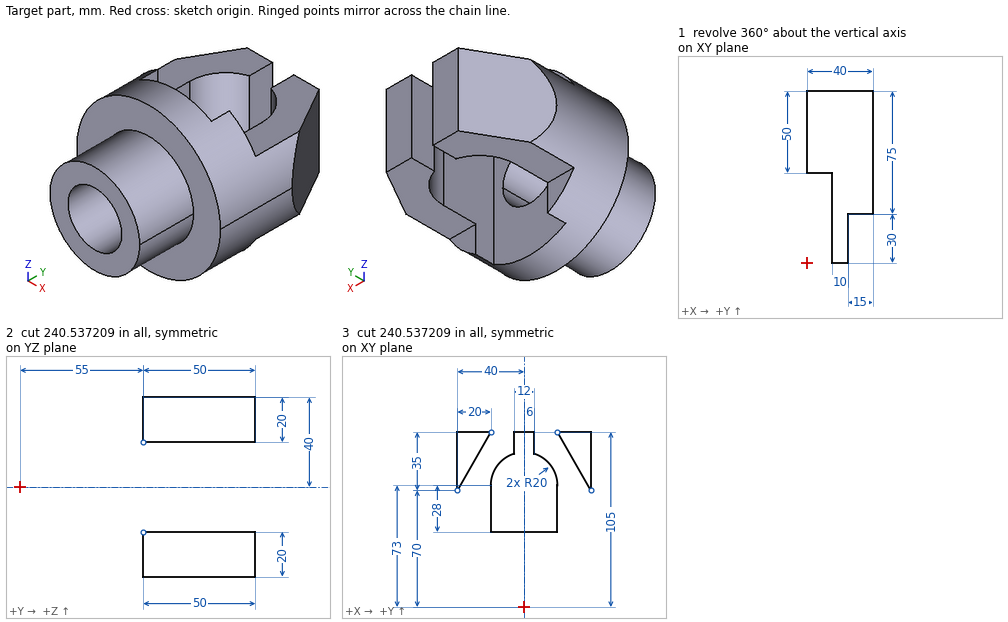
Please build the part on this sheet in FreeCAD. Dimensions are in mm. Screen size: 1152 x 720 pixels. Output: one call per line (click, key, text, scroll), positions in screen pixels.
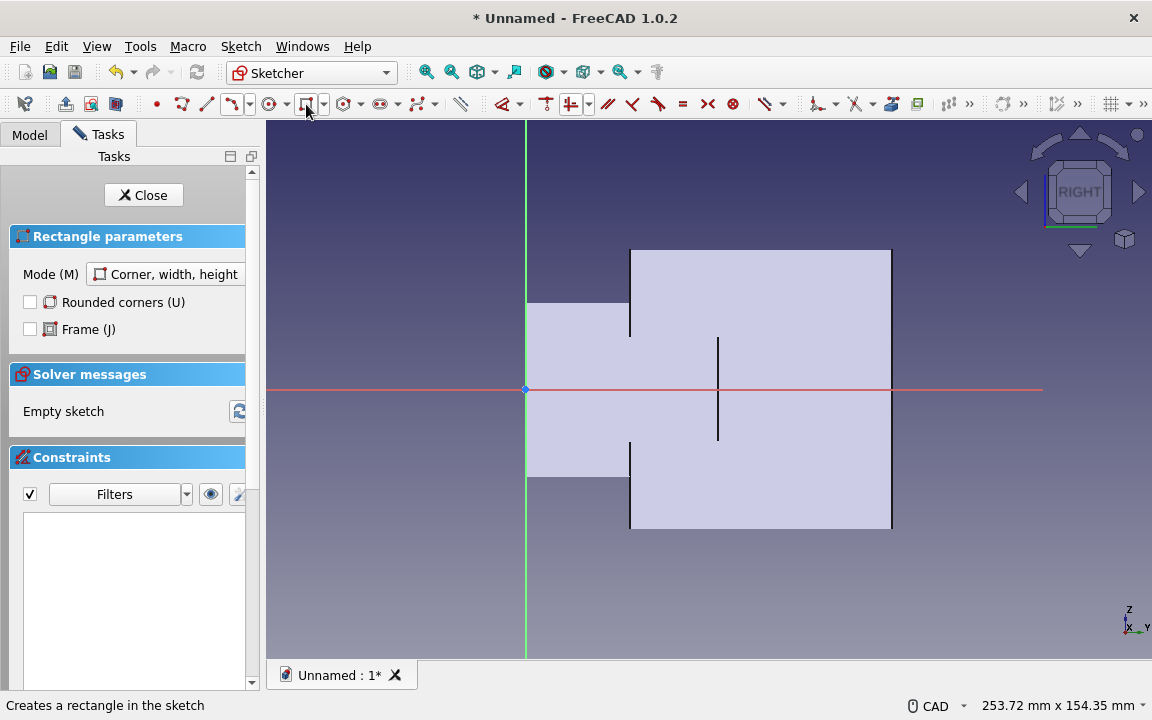
click(718, 250)
move(892, 320)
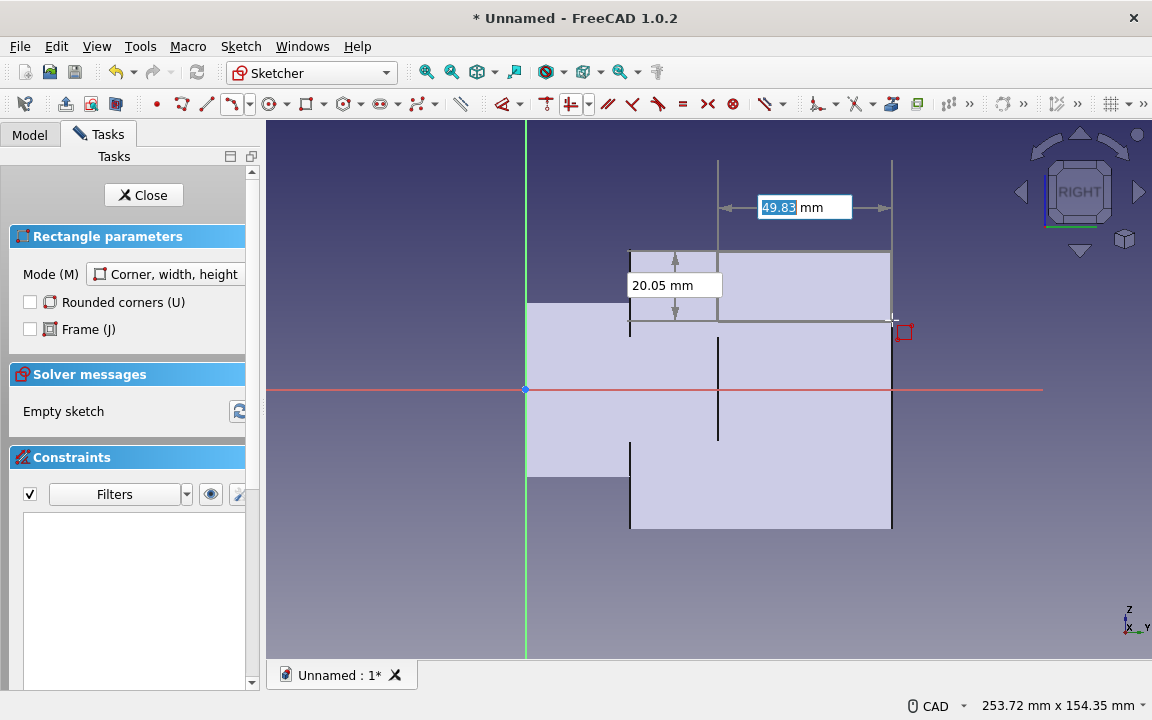
text(50)
key(Tab)
text(20)
key(Return)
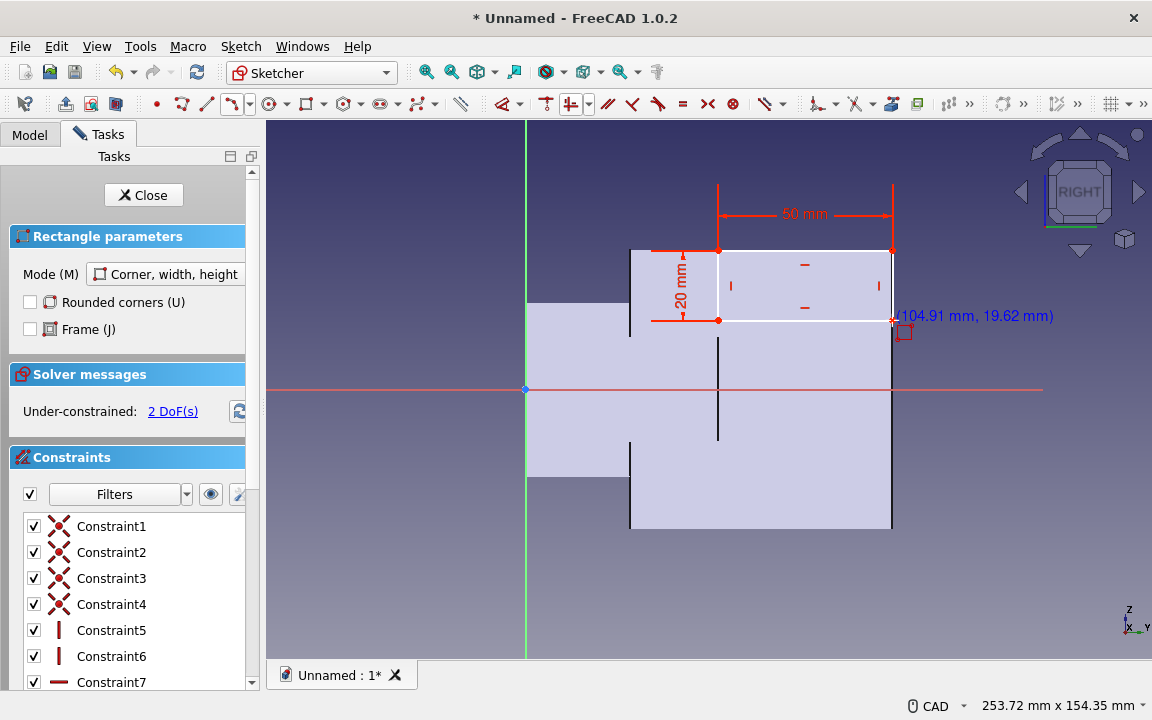
click(718, 459)
move(892, 529)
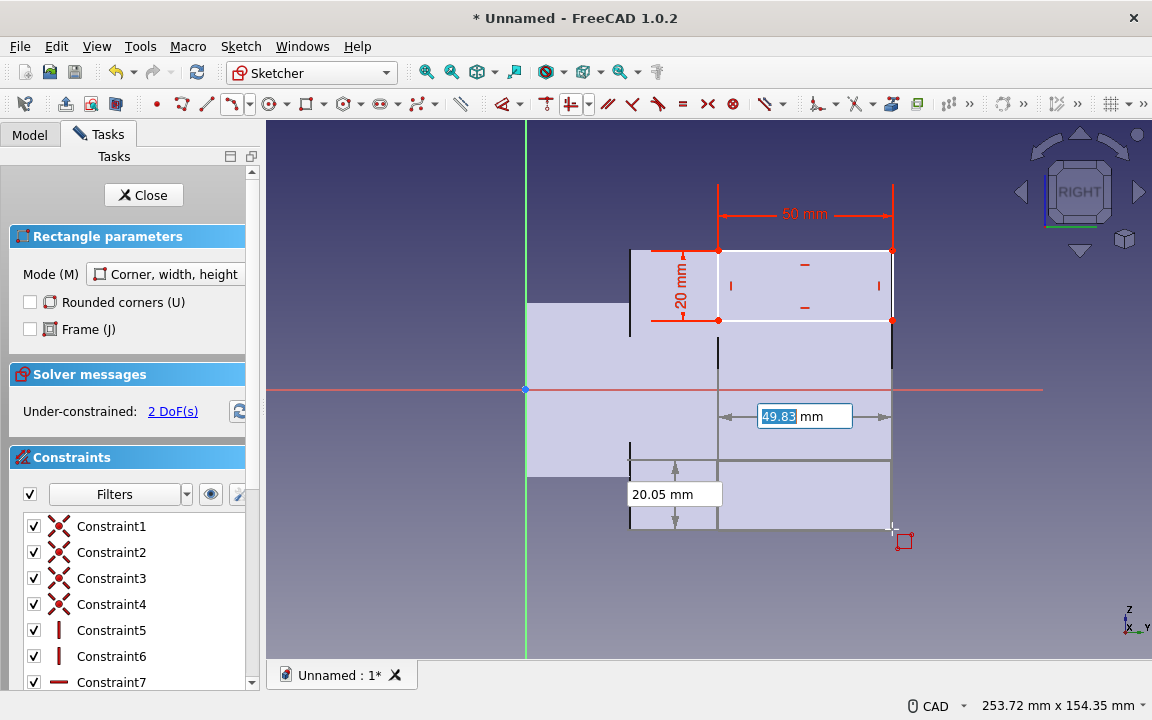
text(50)
key(Tab)
text(20)
key(Return)
key(Escape)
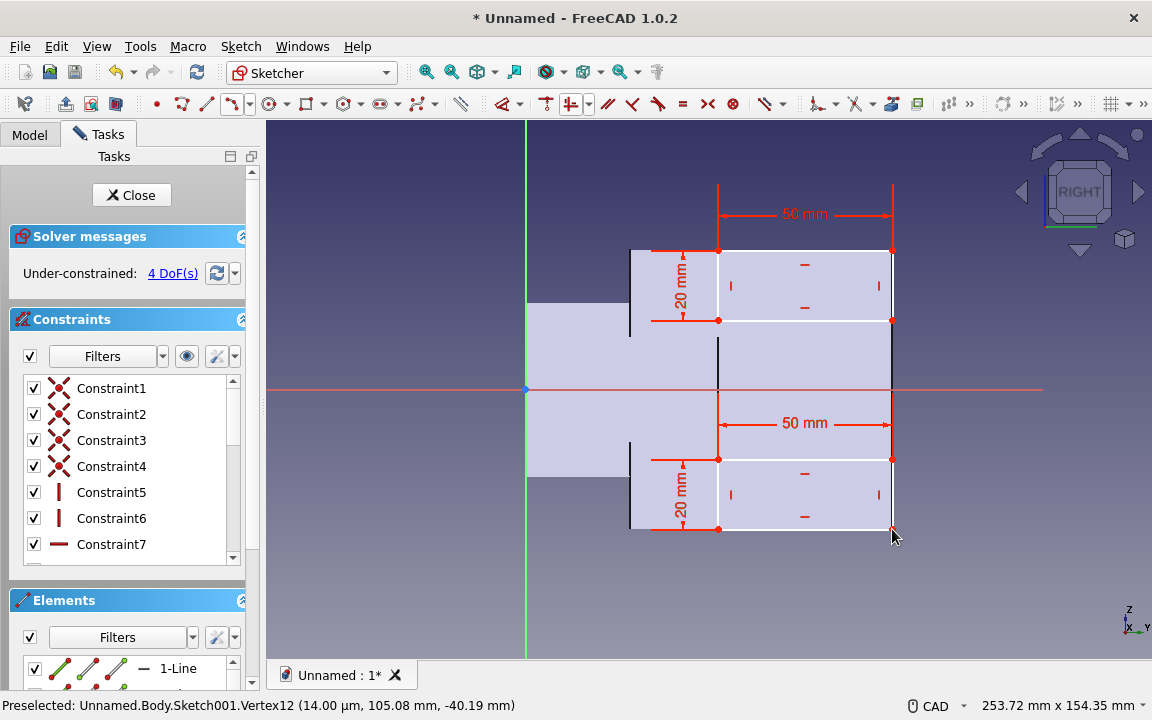
click(718, 321)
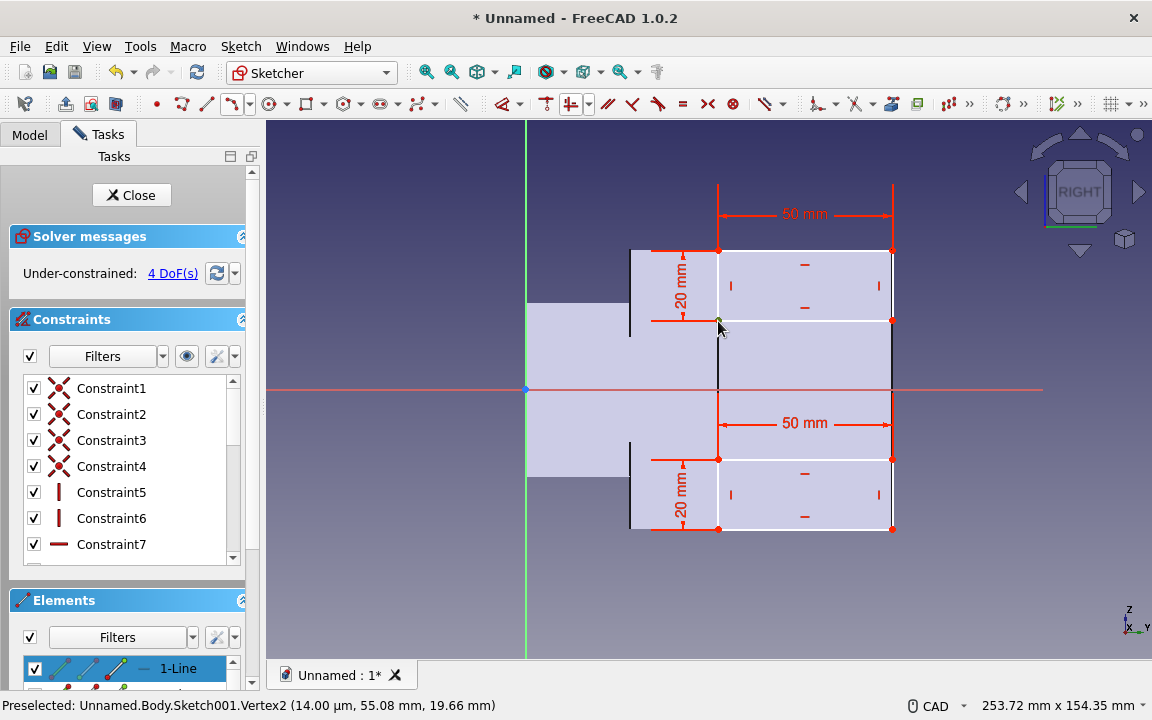
click(718, 460)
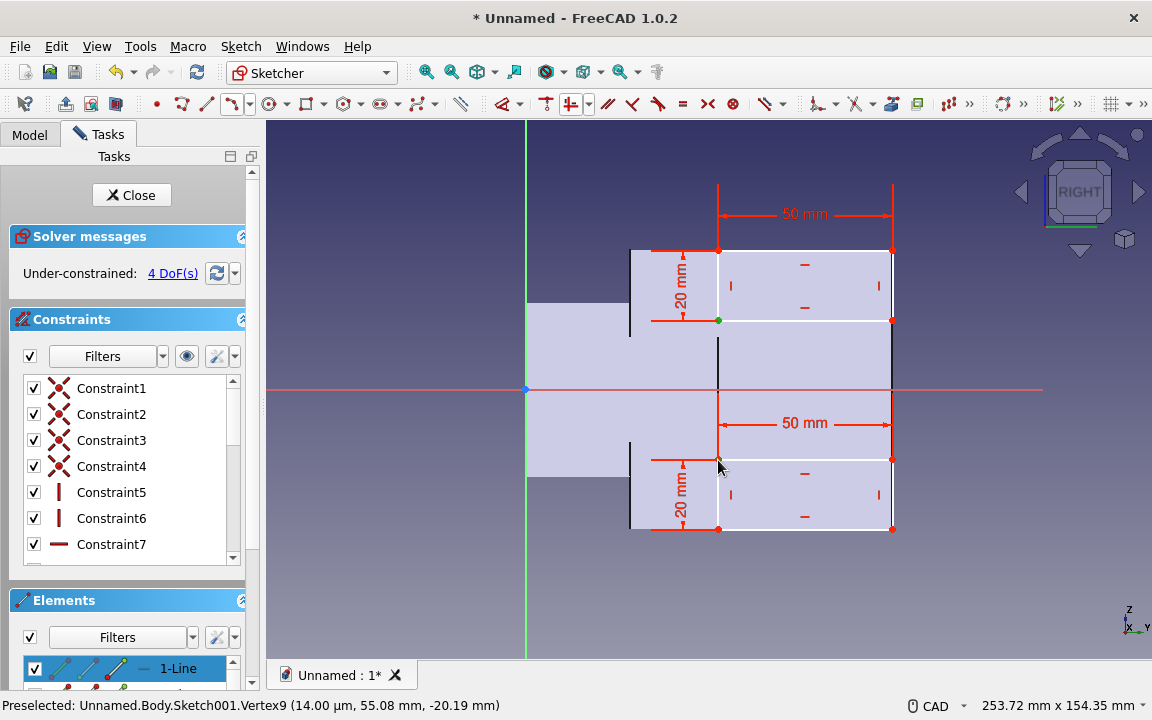
click(344, 390)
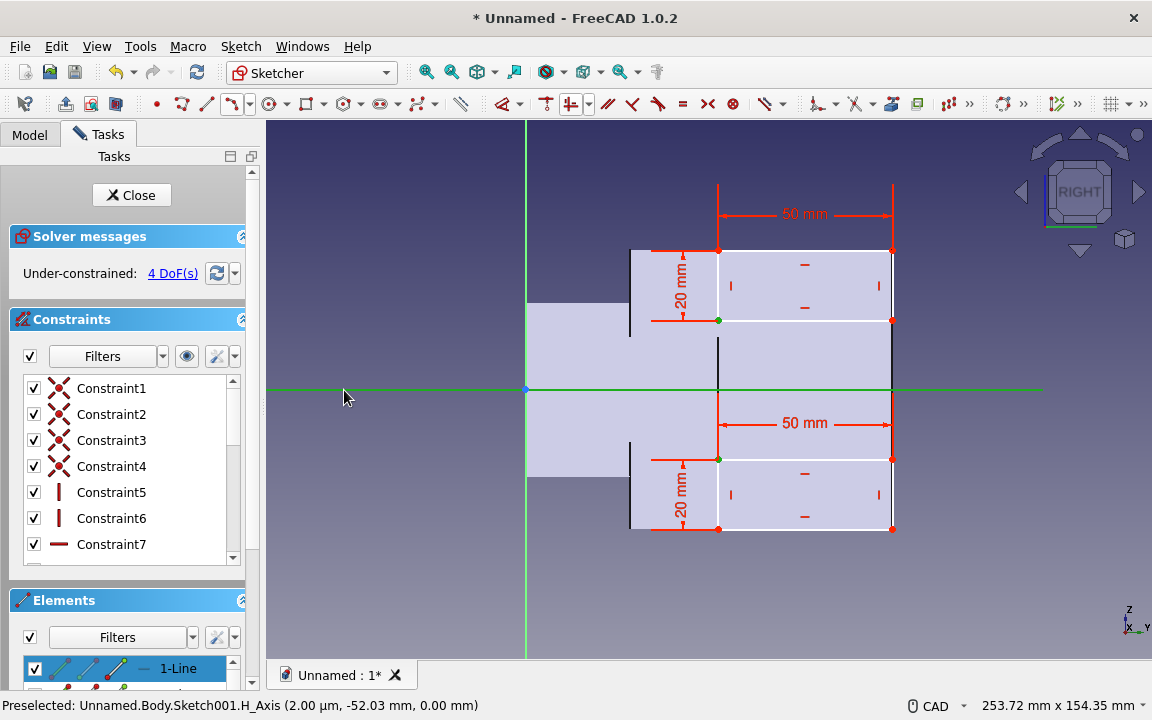
click(708, 104)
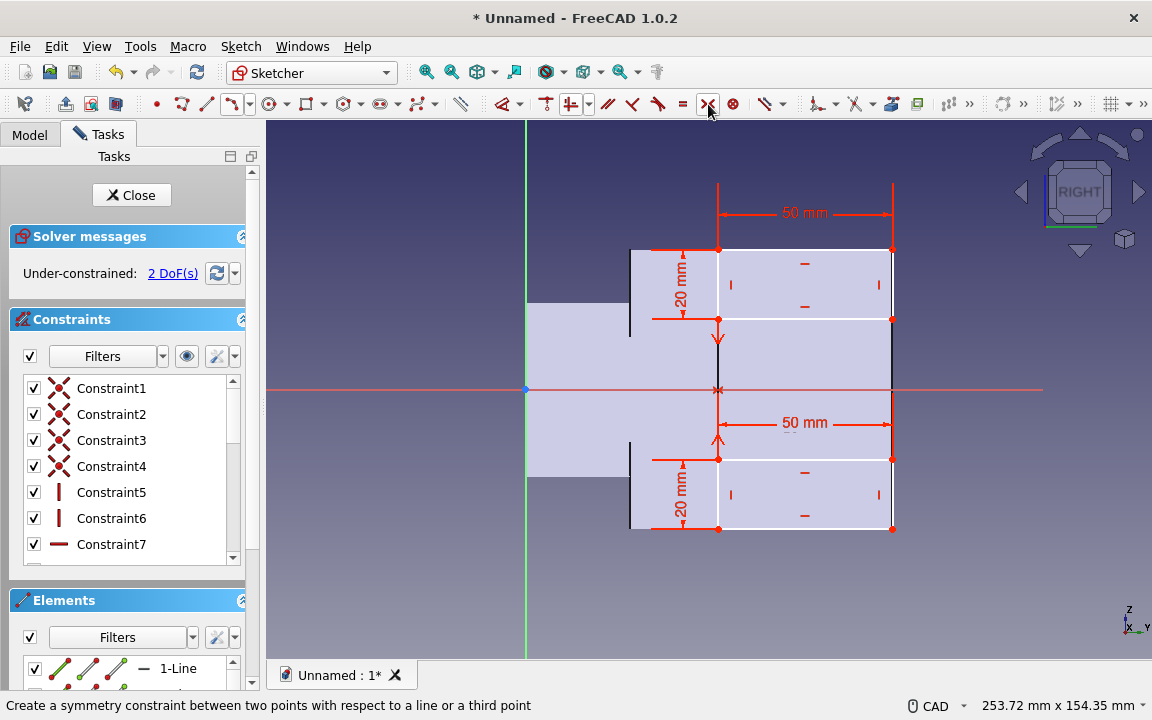
click(502, 104)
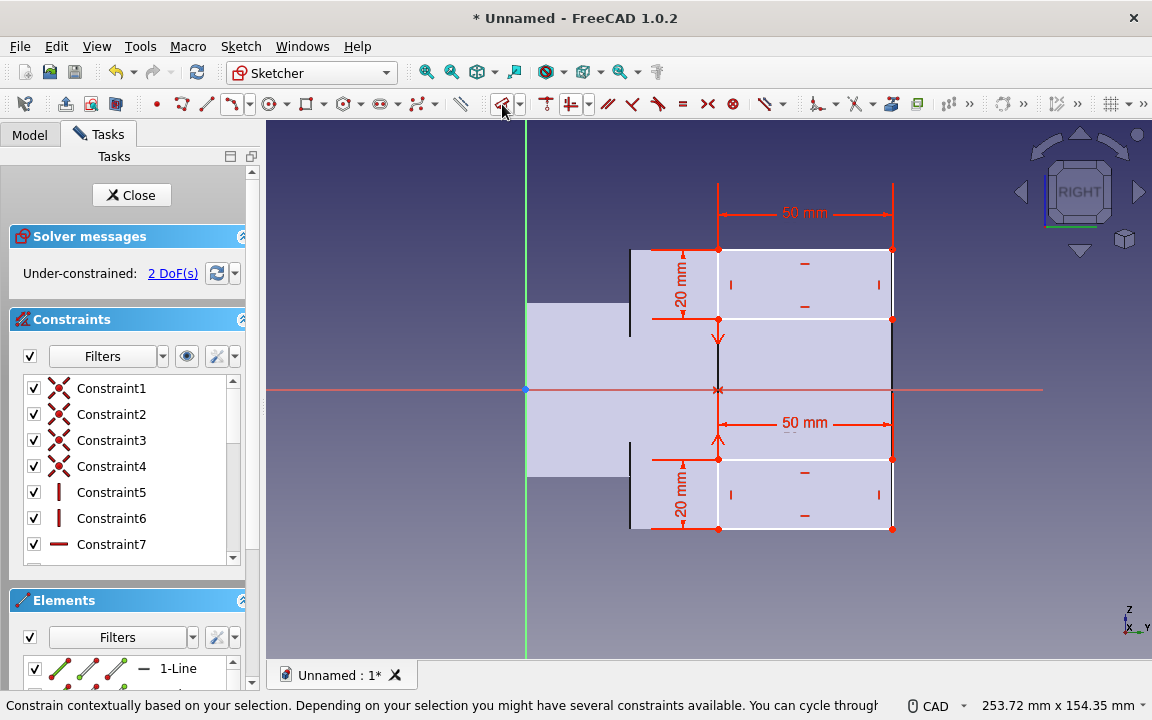
click(718, 250)
click(622, 216)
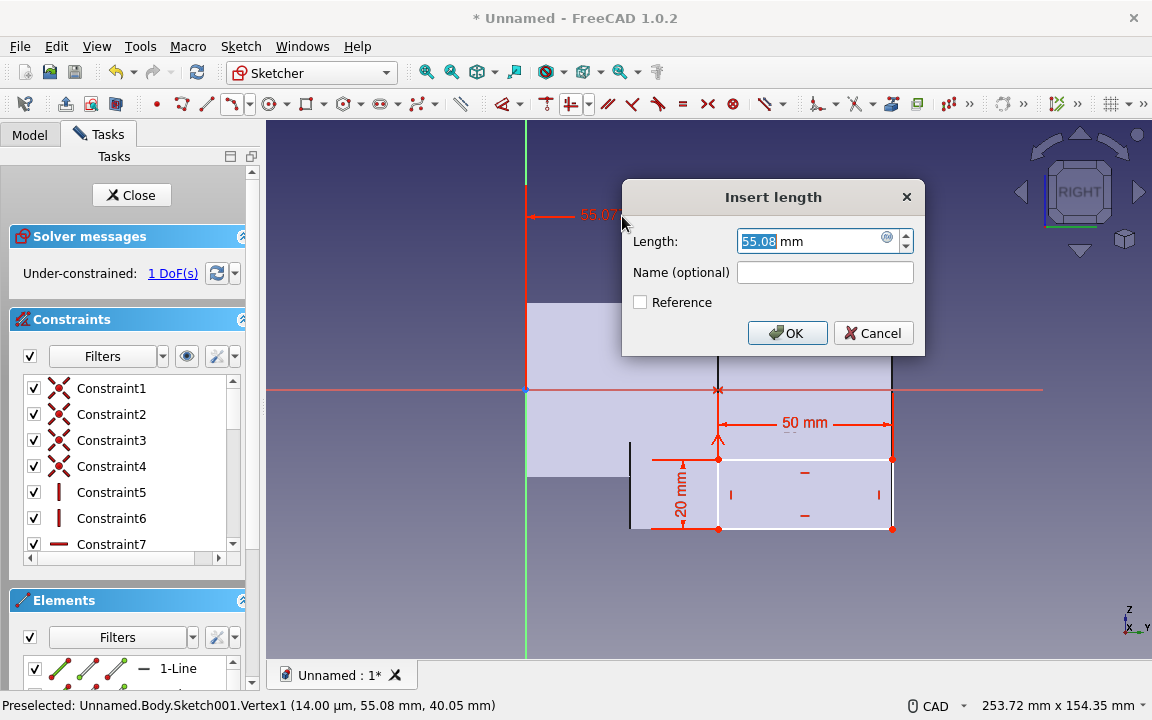
text(55)
key(Return)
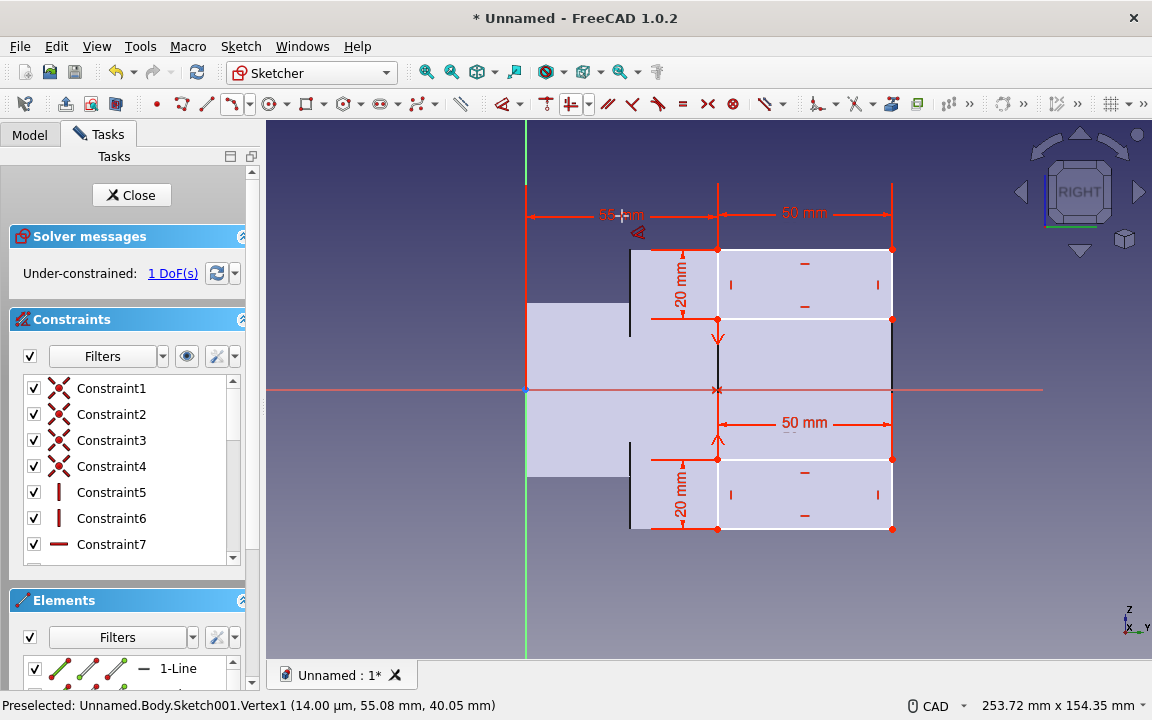
click(718, 250)
click(492, 320)